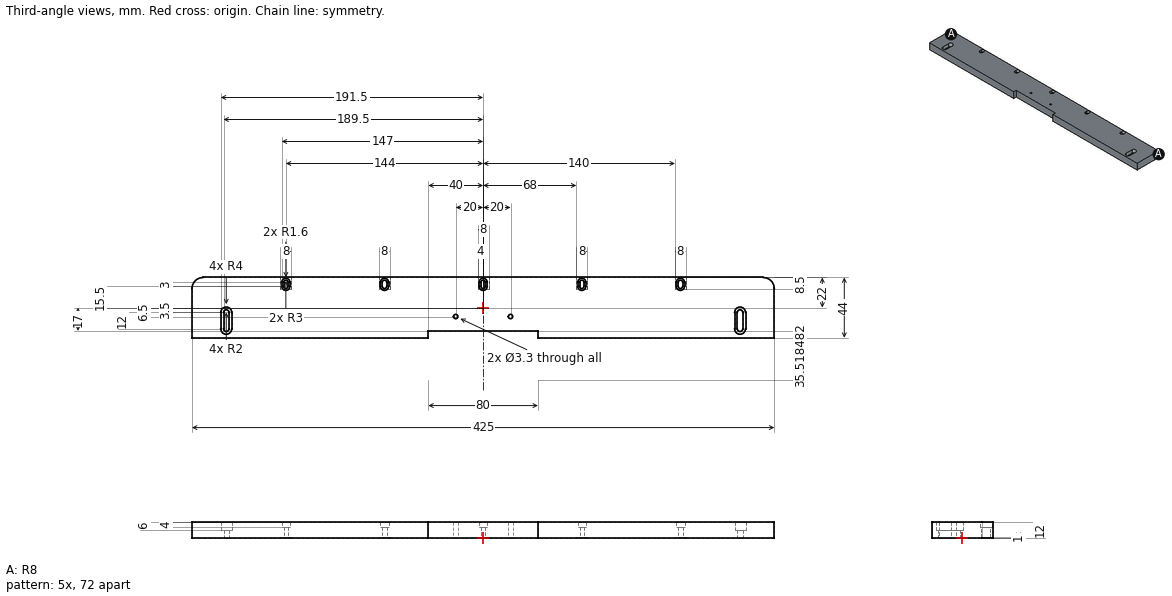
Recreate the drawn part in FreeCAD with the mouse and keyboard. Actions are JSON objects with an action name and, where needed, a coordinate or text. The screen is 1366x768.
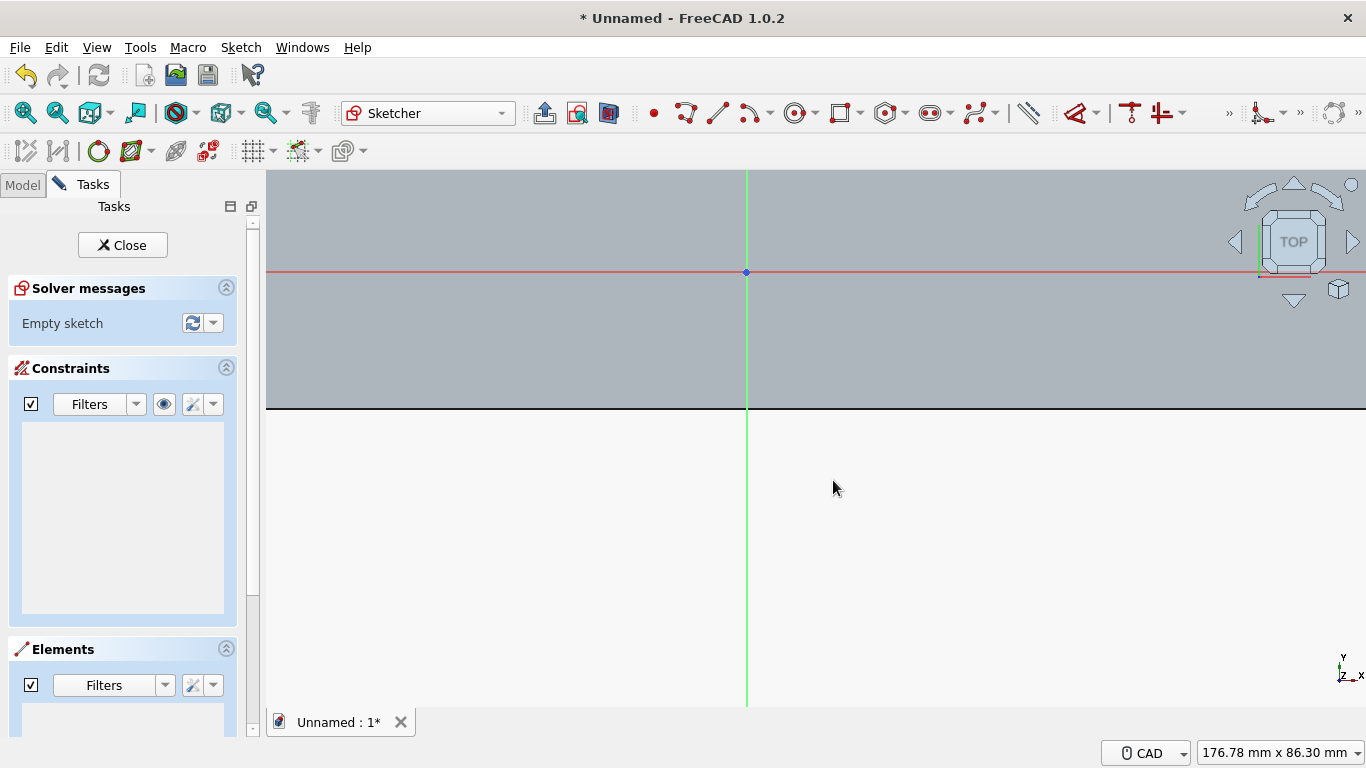
{"action": "left_click", "coordinate": [840, 114]}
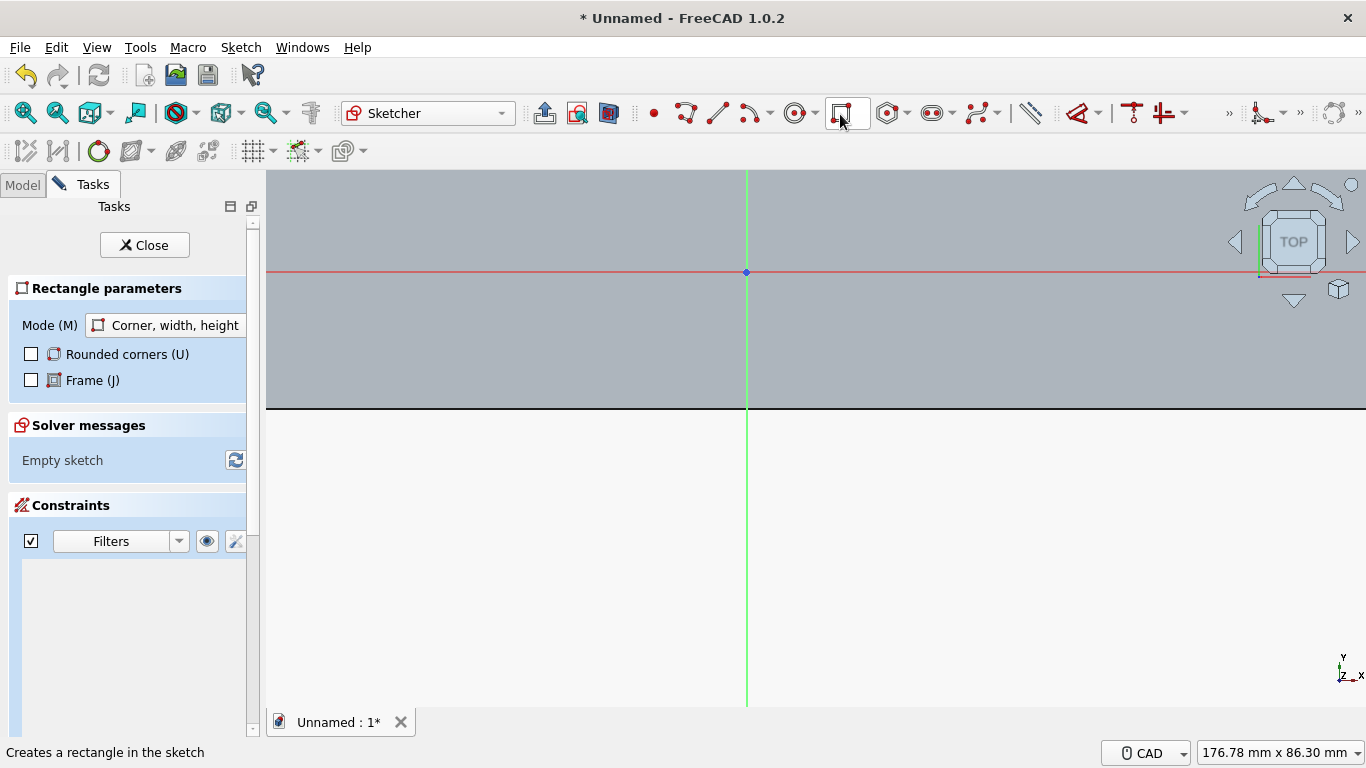
{"action": "left_click", "coordinate": [498, 378]}
{"action": "mouse_move", "coordinate": [996, 599]}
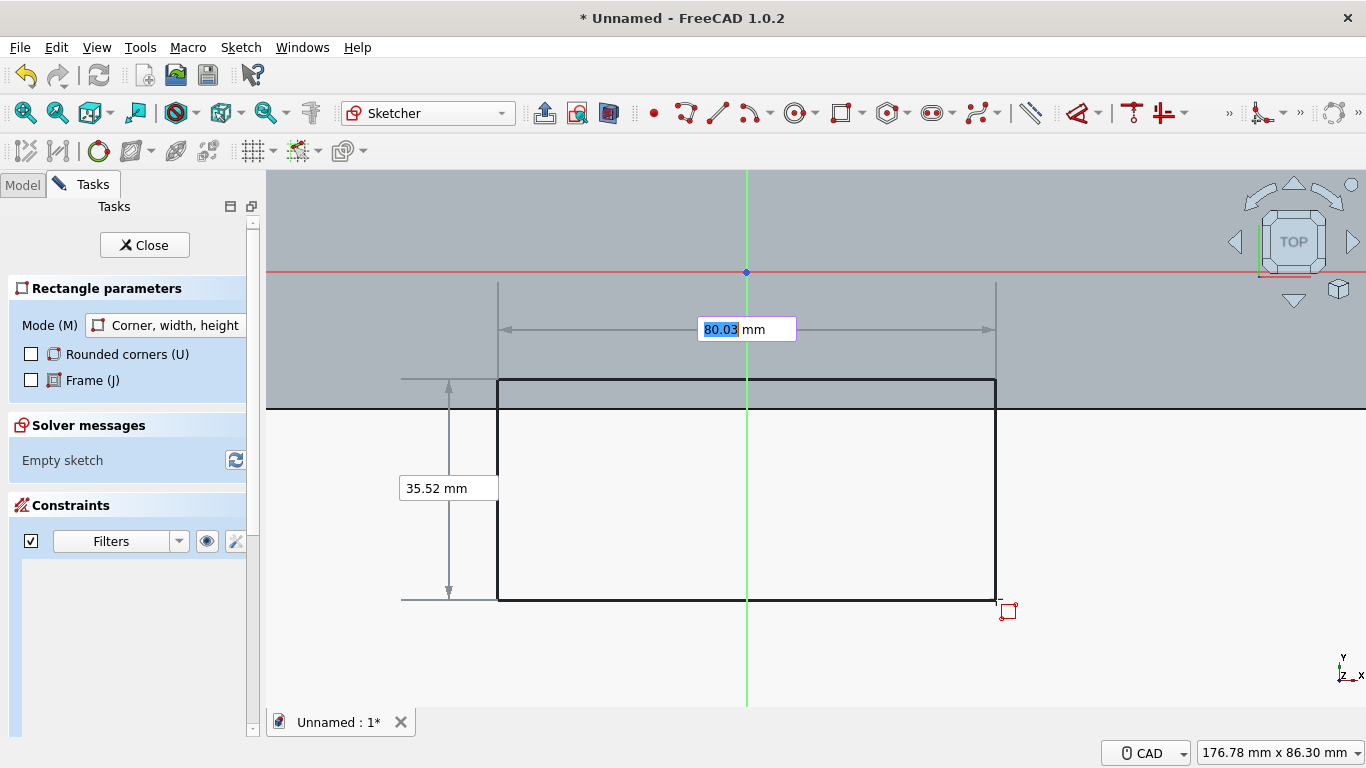
{"action": "type", "text": "80"}
{"action": "key", "text": "Tab"}
{"action": "type", "text": "35.518482"}
{"action": "key", "text": "Return"}
{"action": "key", "text": "Escape"}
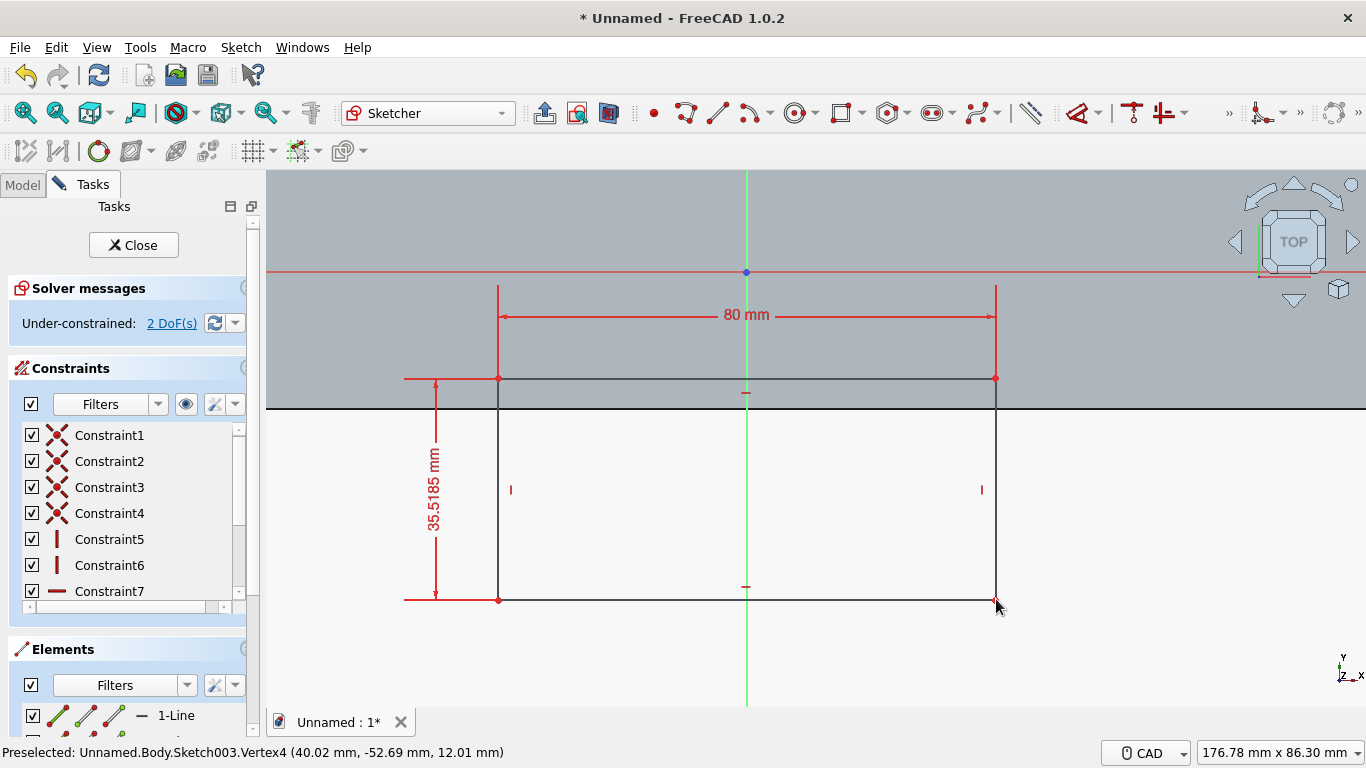
{"action": "left_click", "coordinate": [1078, 114]}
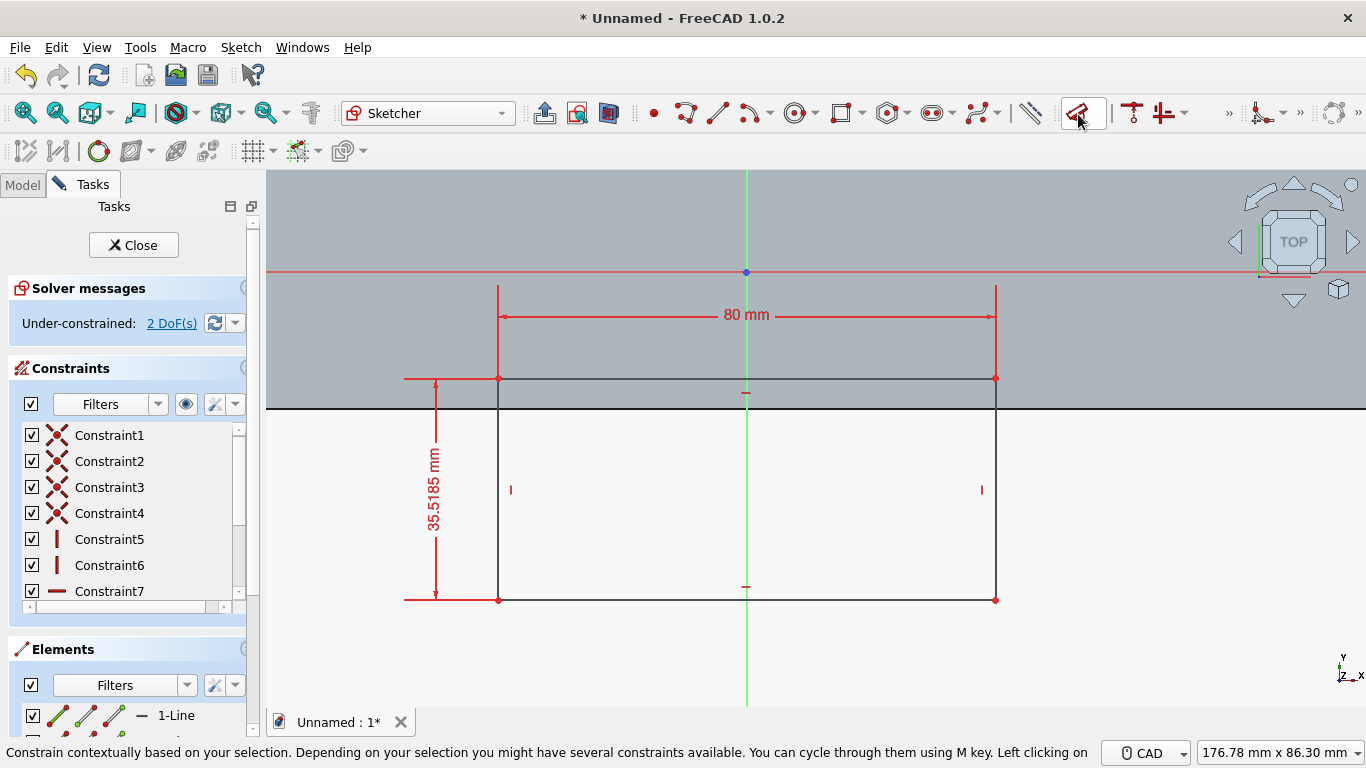
{"action": "left_click", "coordinate": [498, 379]}
{"action": "left_click", "coordinate": [622, 238]}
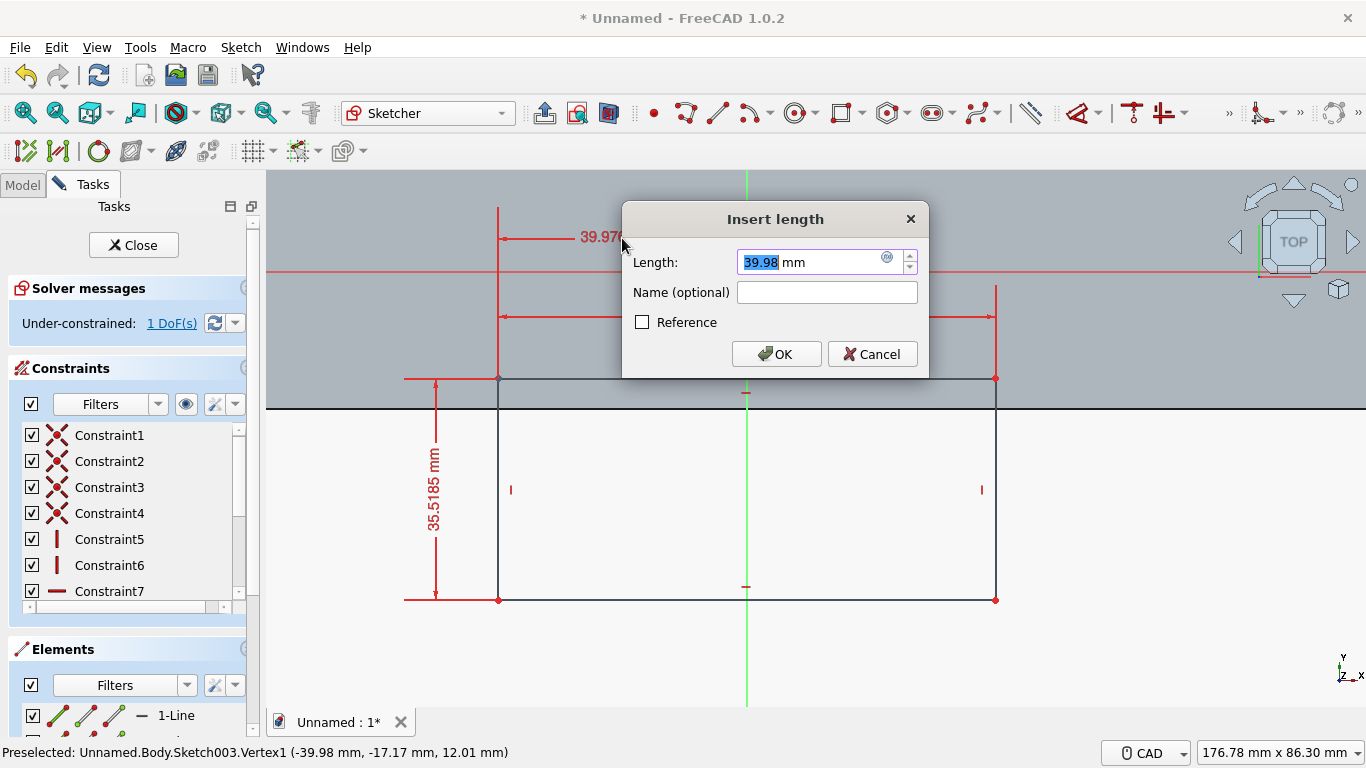
{"action": "type", "text": "40"}
{"action": "key", "text": "Return"}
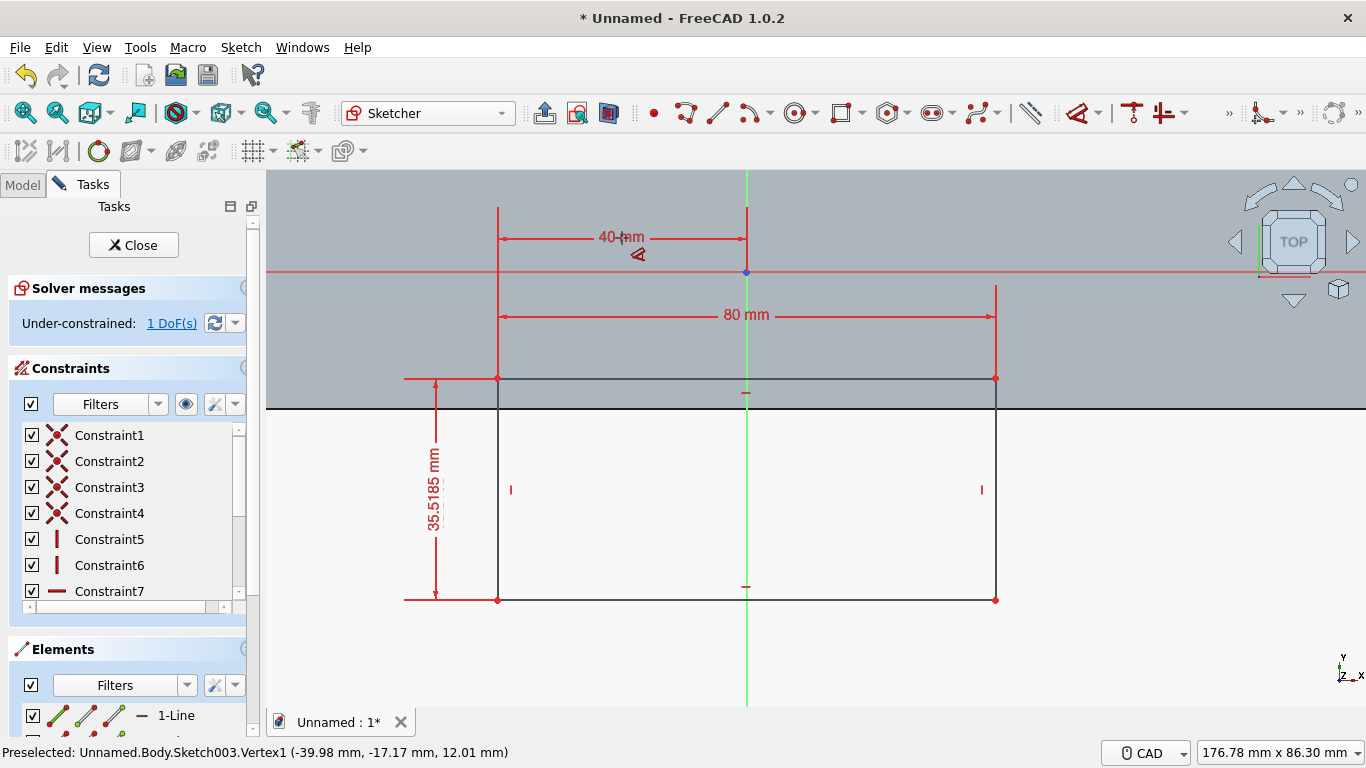
{"action": "left_click", "coordinate": [498, 379]}
{"action": "left_click", "coordinate": [464, 326]}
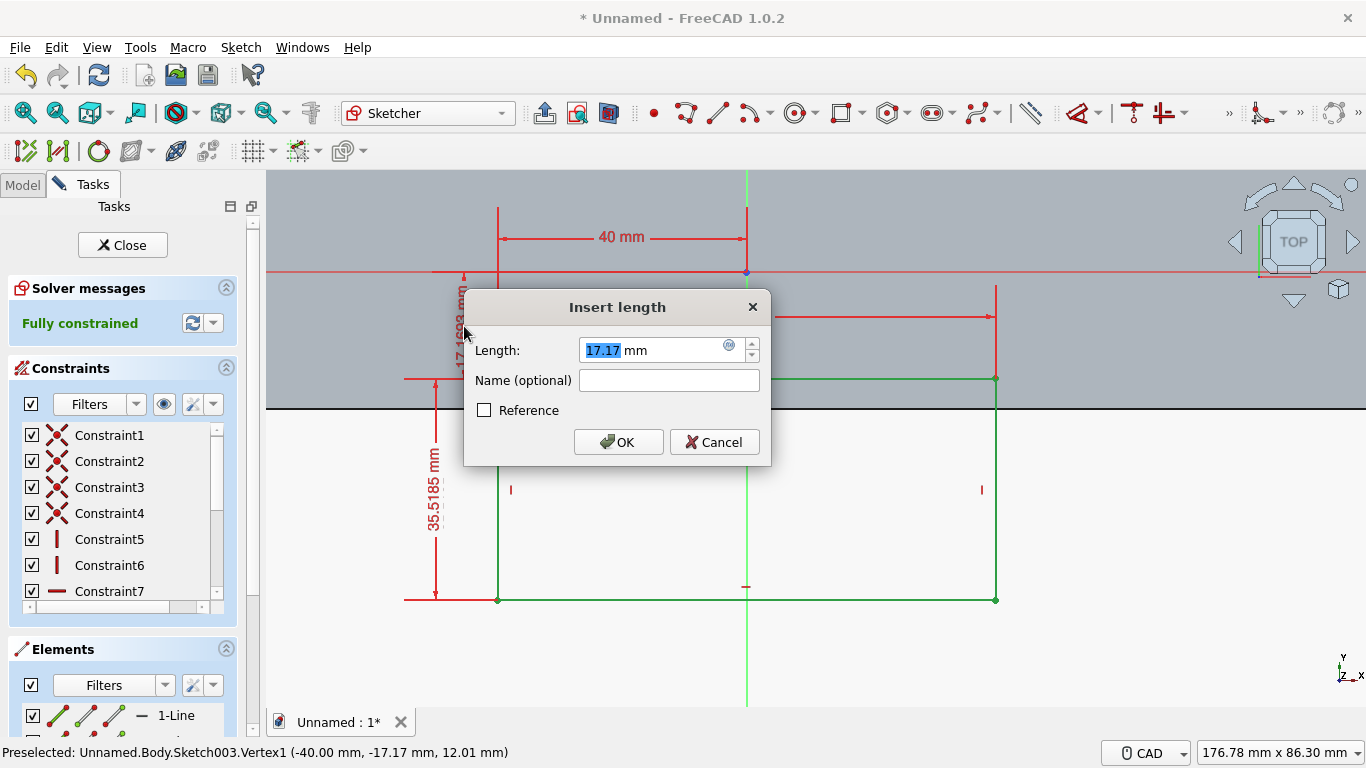
{"action": "type", "text": "17"}
{"action": "key", "text": "Return"}
{"action": "key", "text": "Escape"}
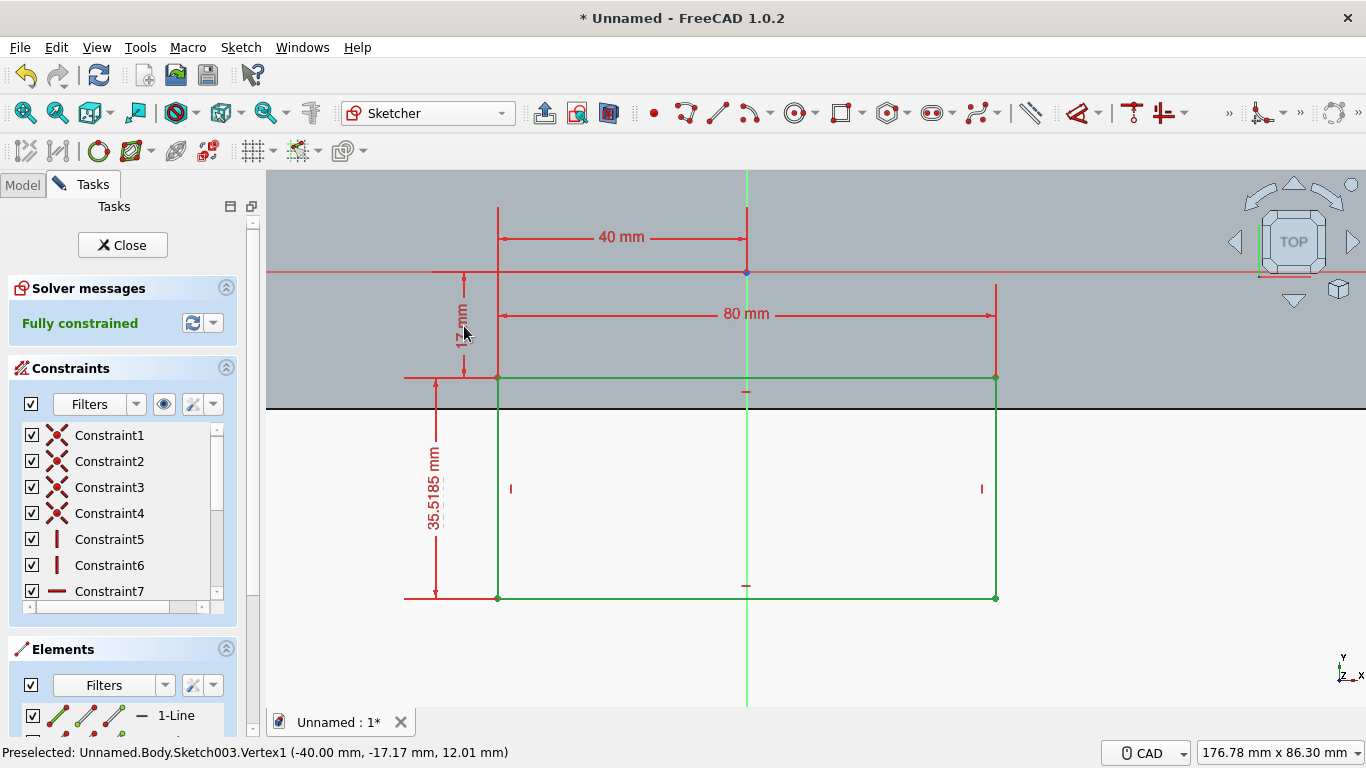
{"action": "left_click", "coordinate": [123, 245]}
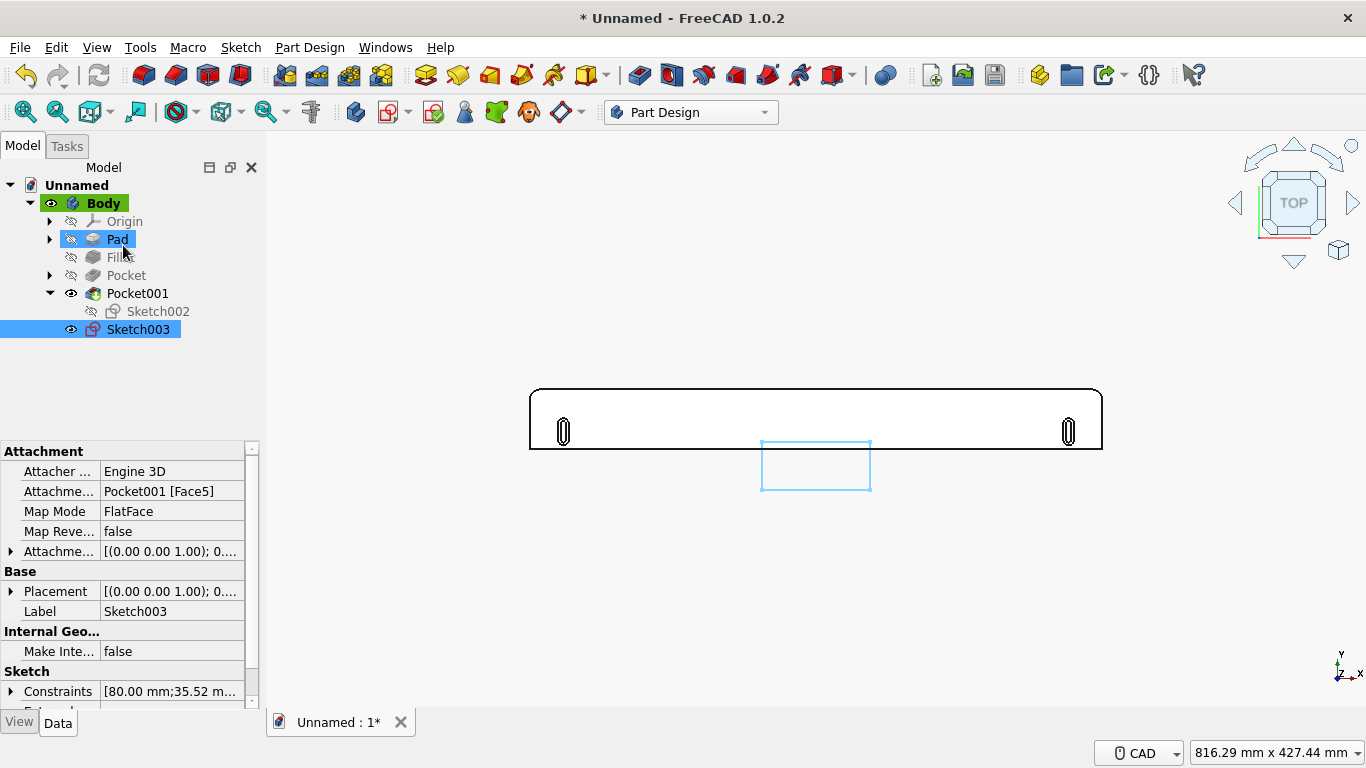
{"action": "left_click", "coordinate": [640, 76]}